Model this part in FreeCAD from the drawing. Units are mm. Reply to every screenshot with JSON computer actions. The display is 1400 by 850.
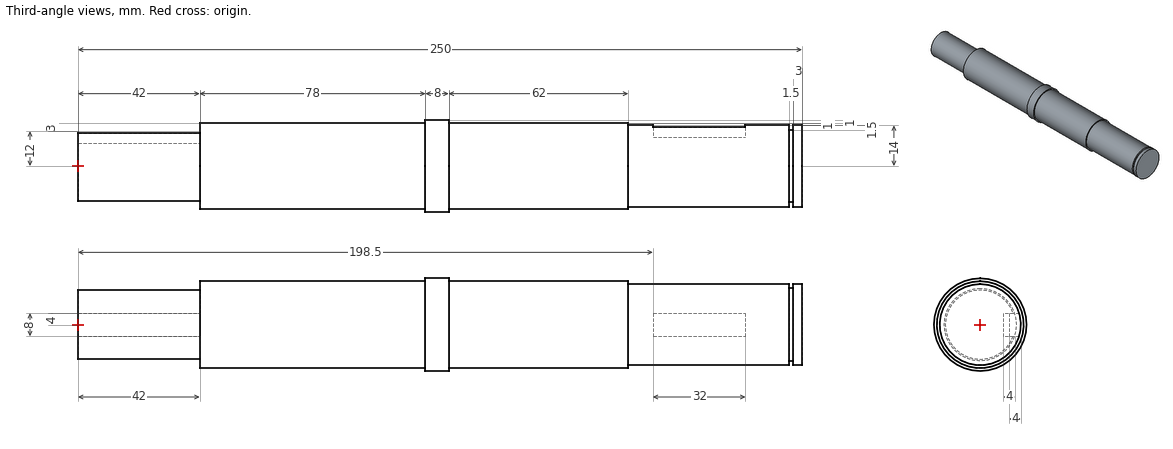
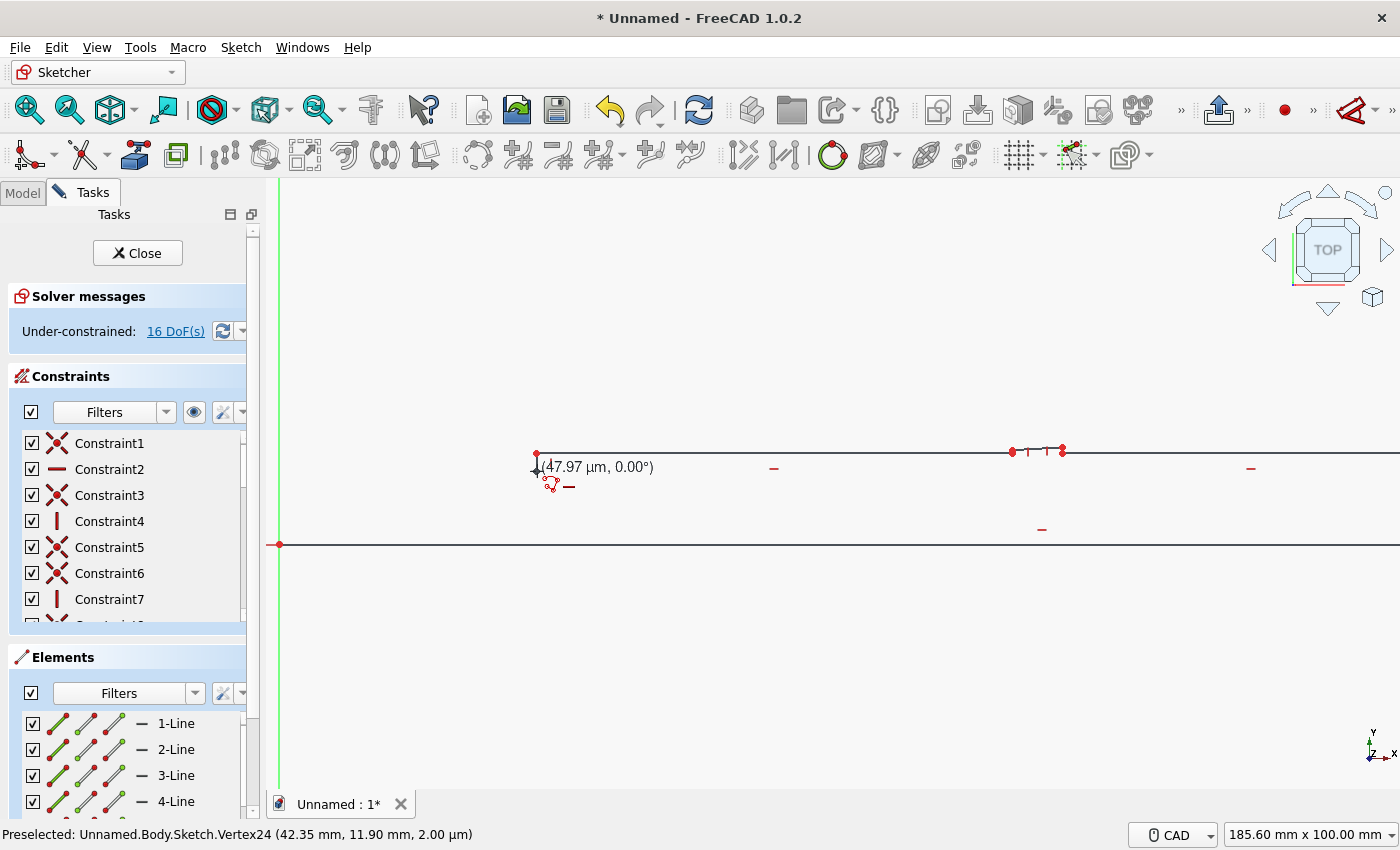
{"action": "scroll", "coordinate": [537, 473], "scroll_direction": "down", "scroll_amount": 4}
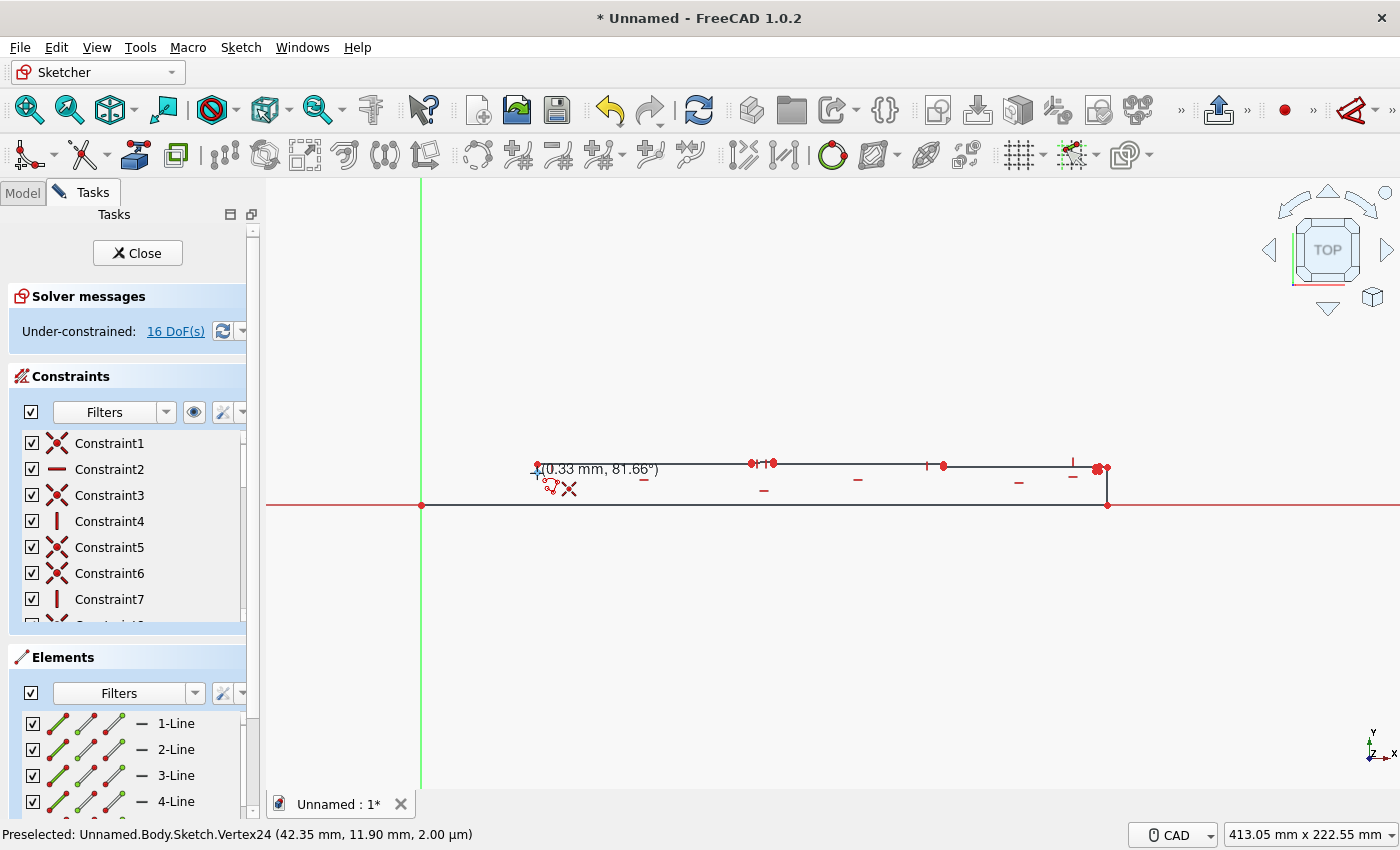
{"action": "left_click", "coordinate": [430, 472]}
{"action": "left_click", "coordinate": [421, 505]}
{"action": "key", "text": "Escape"}
{"action": "key", "text": "Escape"}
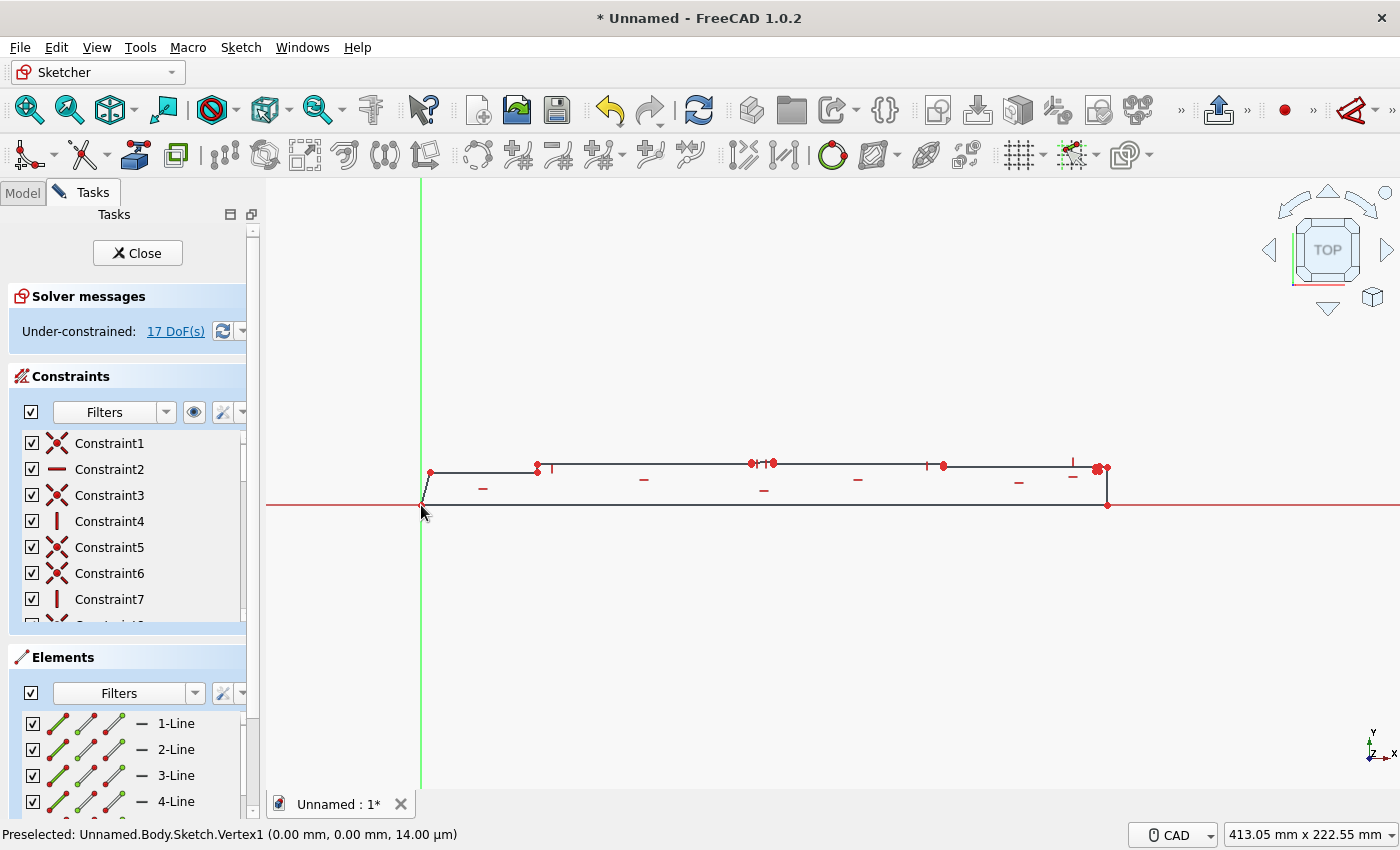
{"action": "scroll", "coordinate": [1103, 467], "scroll_direction": "up", "scroll_amount": 7}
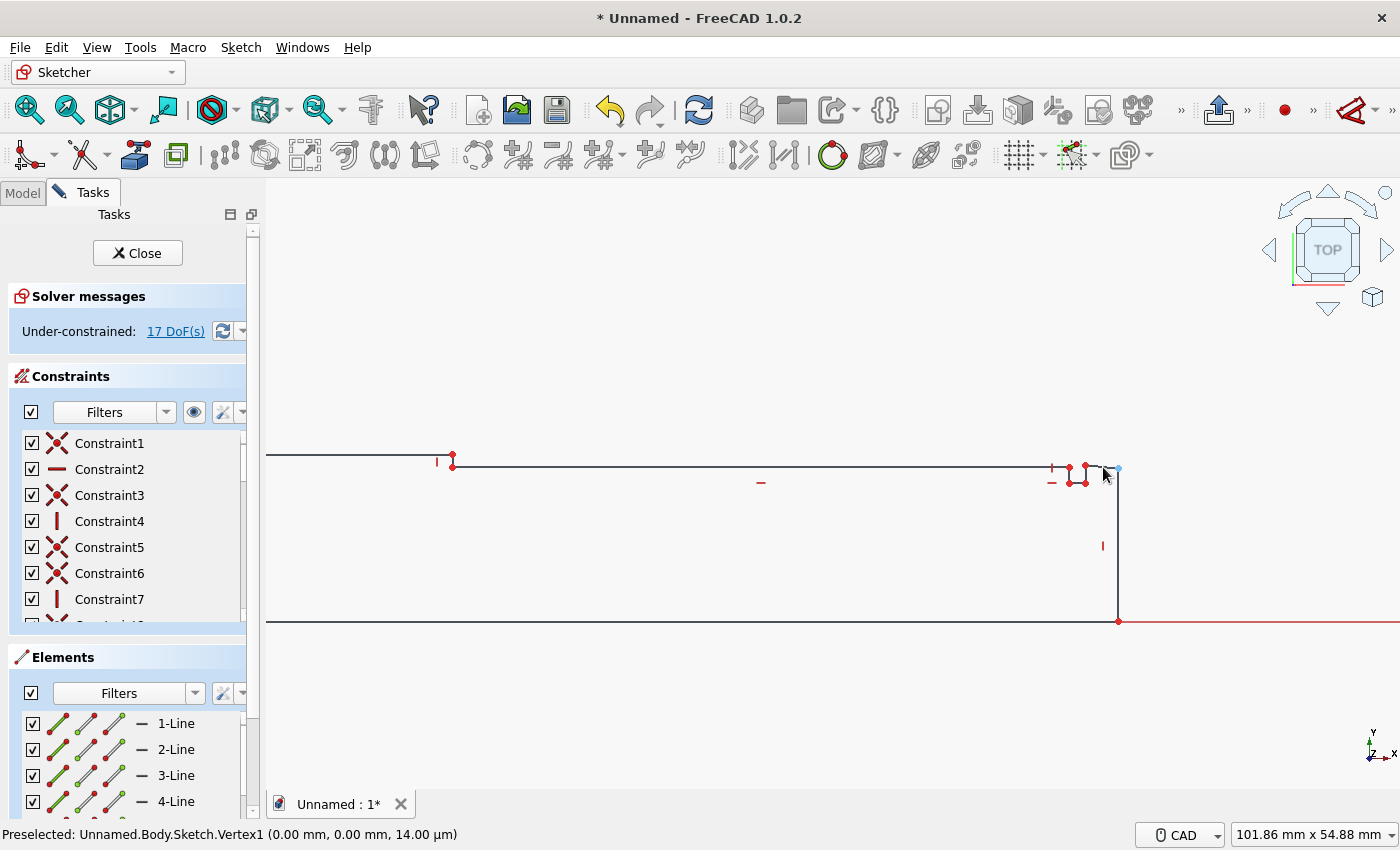
{"action": "left_click", "coordinate": [1102, 467]}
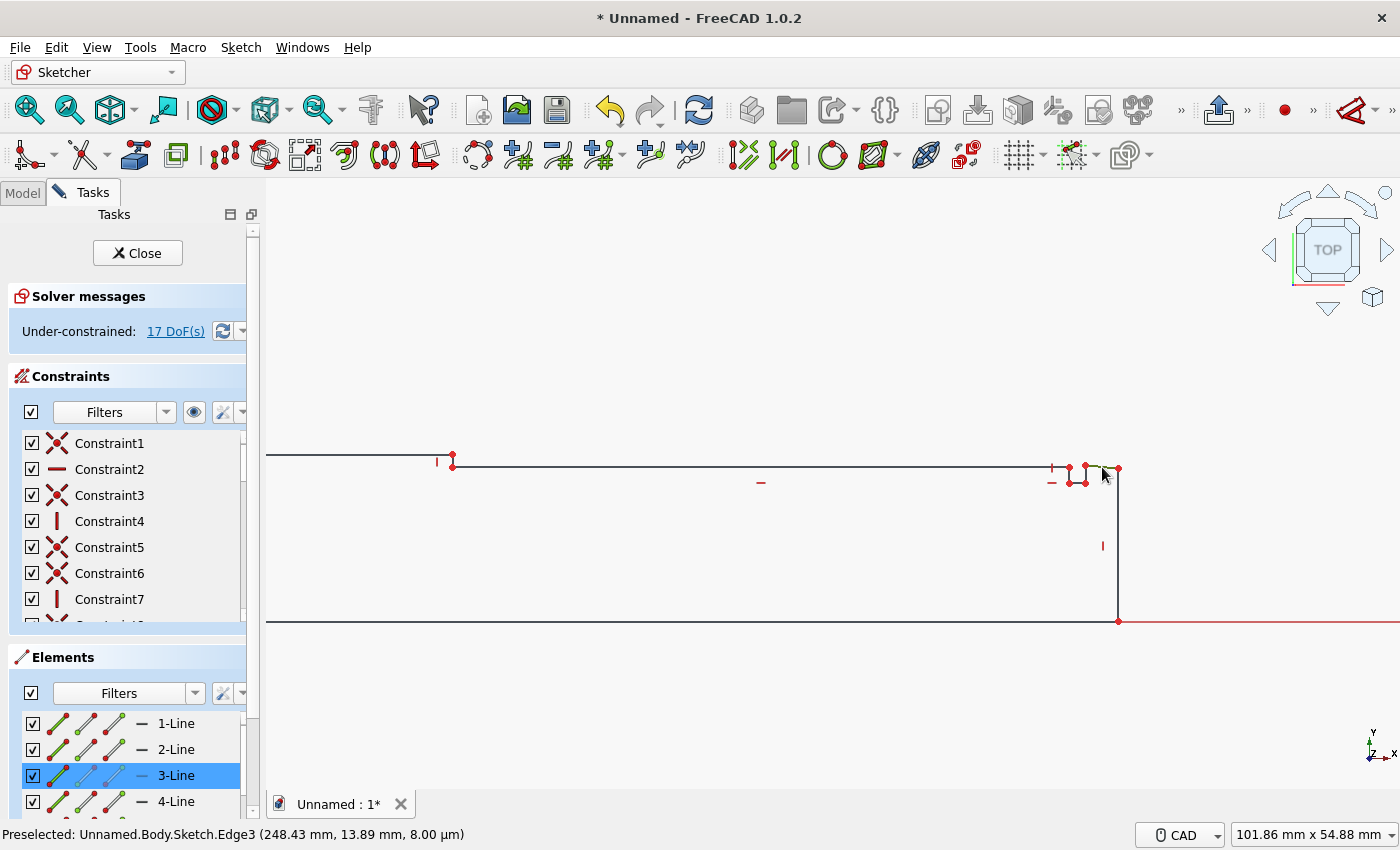
{"action": "key", "text": "h"}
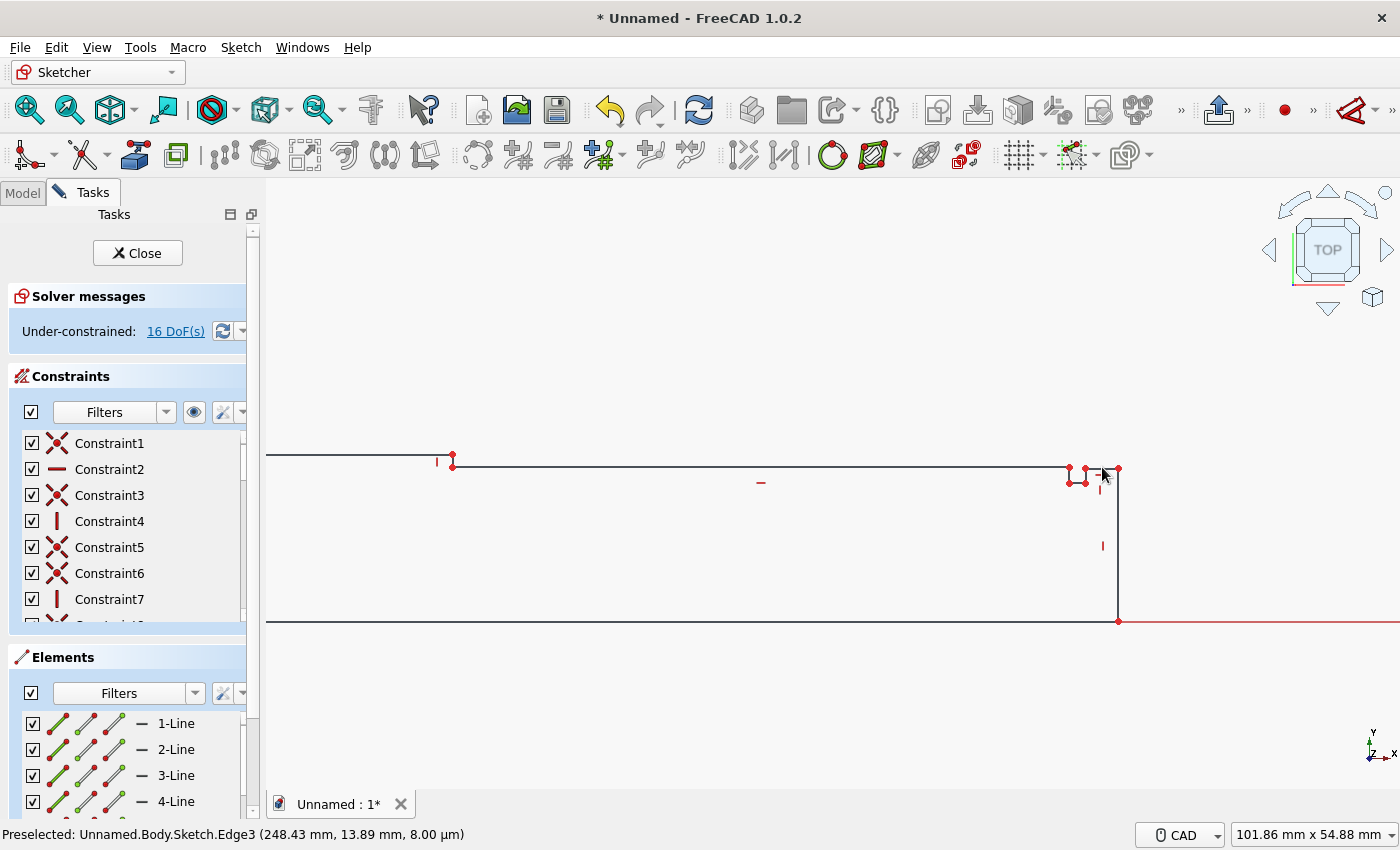
{"action": "scroll", "coordinate": [1104, 467], "scroll_direction": "down", "scroll_amount": 7}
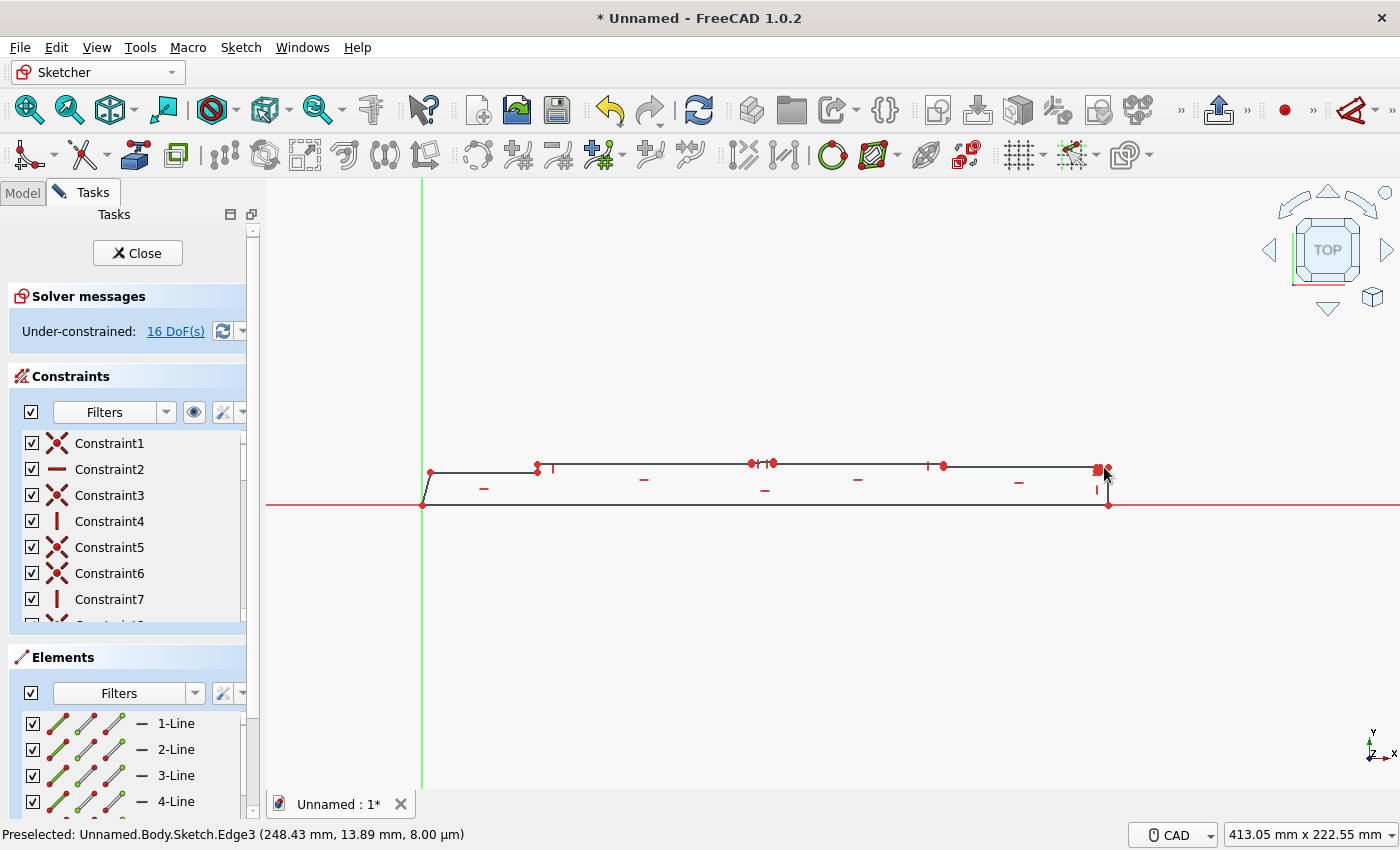
{"action": "scroll", "coordinate": [767, 462], "scroll_direction": "up", "scroll_amount": 4}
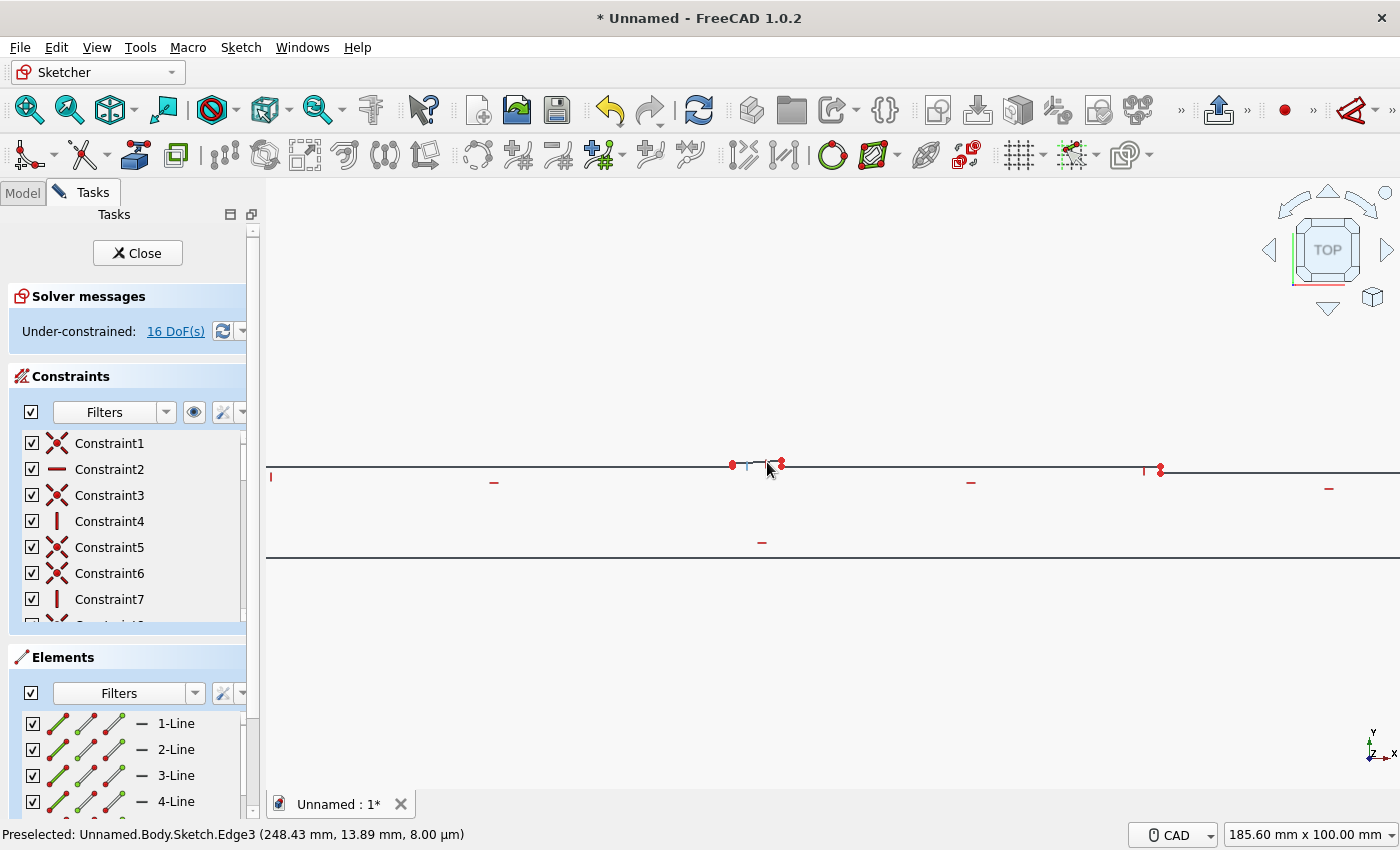
{"action": "left_click", "coordinate": [757, 462]}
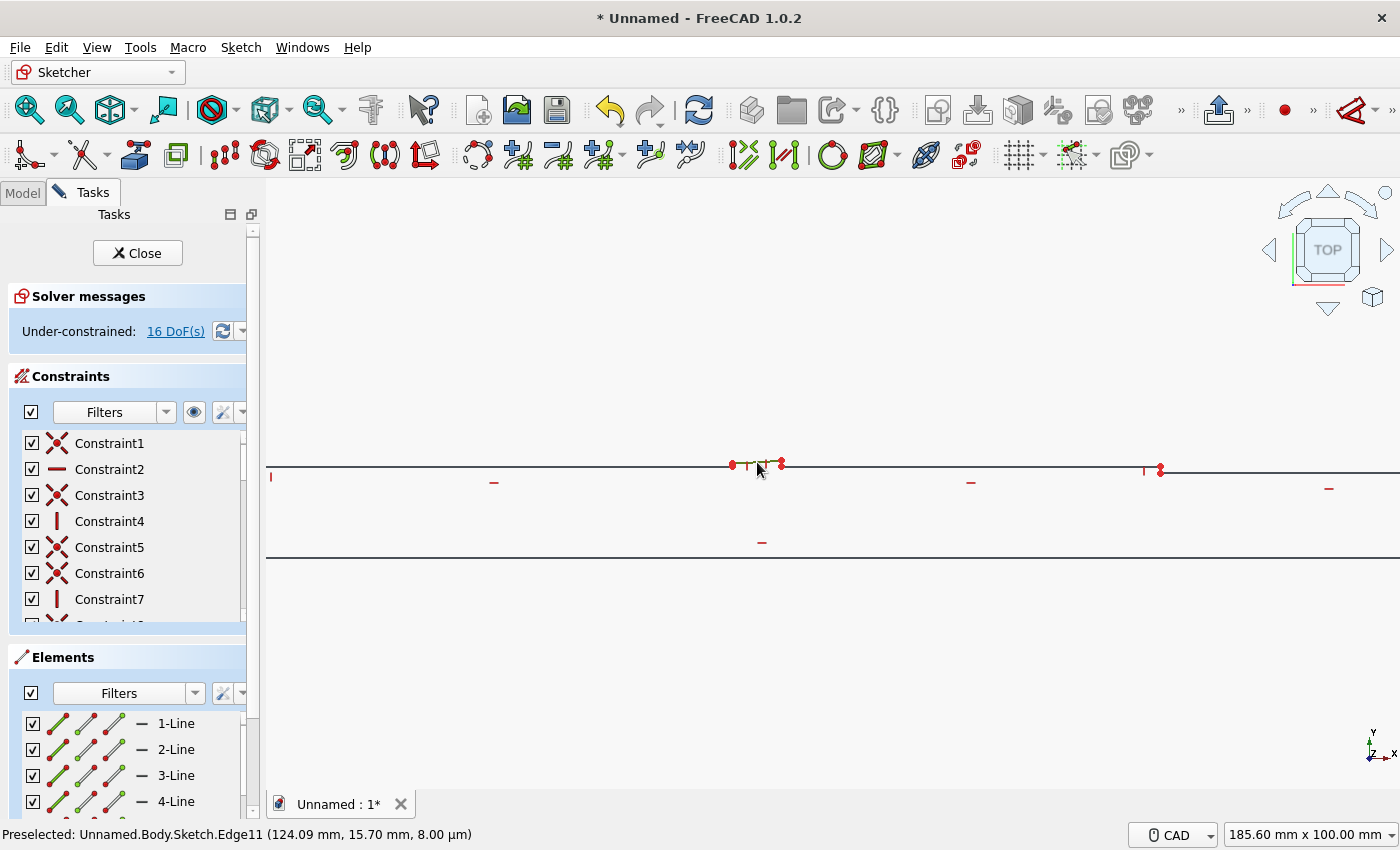
{"action": "key", "text": "h"}